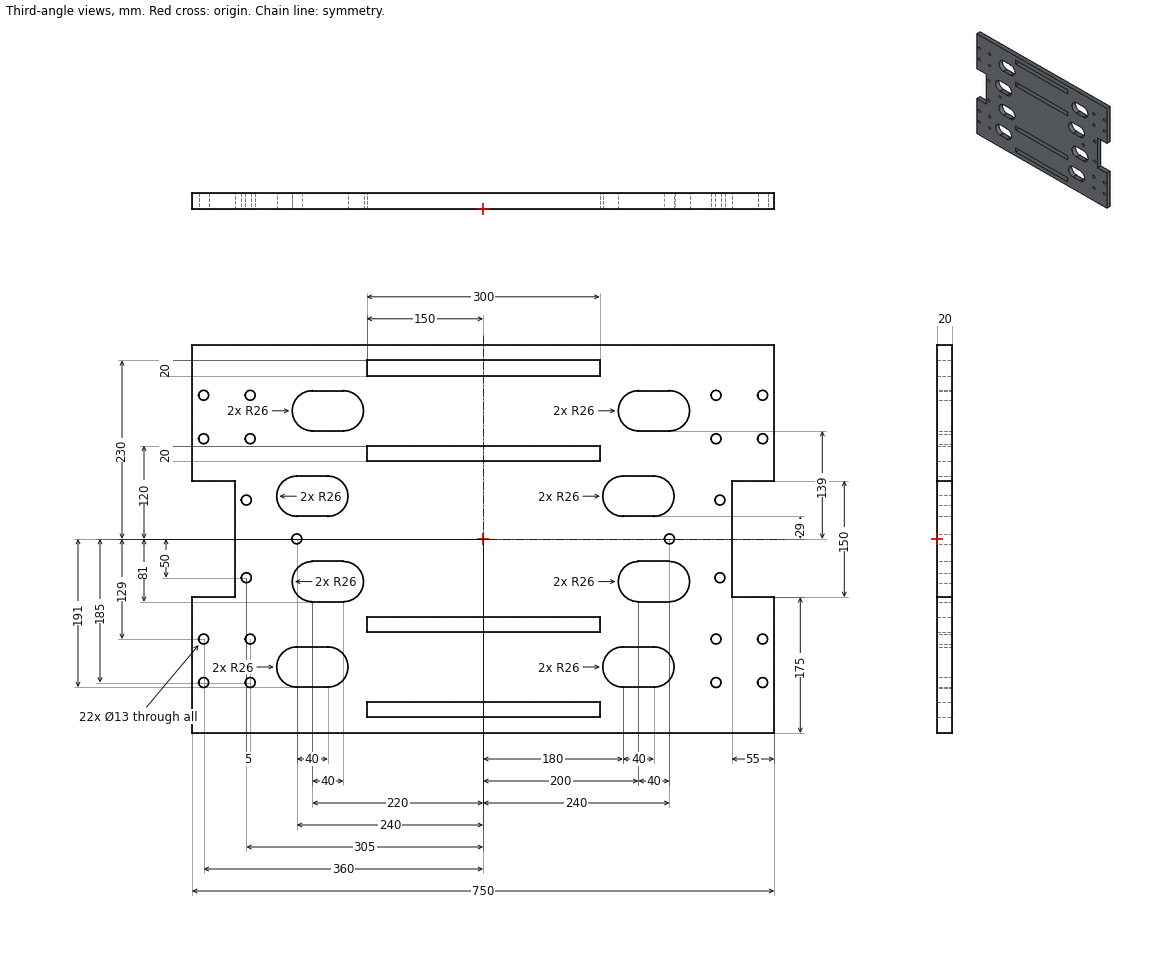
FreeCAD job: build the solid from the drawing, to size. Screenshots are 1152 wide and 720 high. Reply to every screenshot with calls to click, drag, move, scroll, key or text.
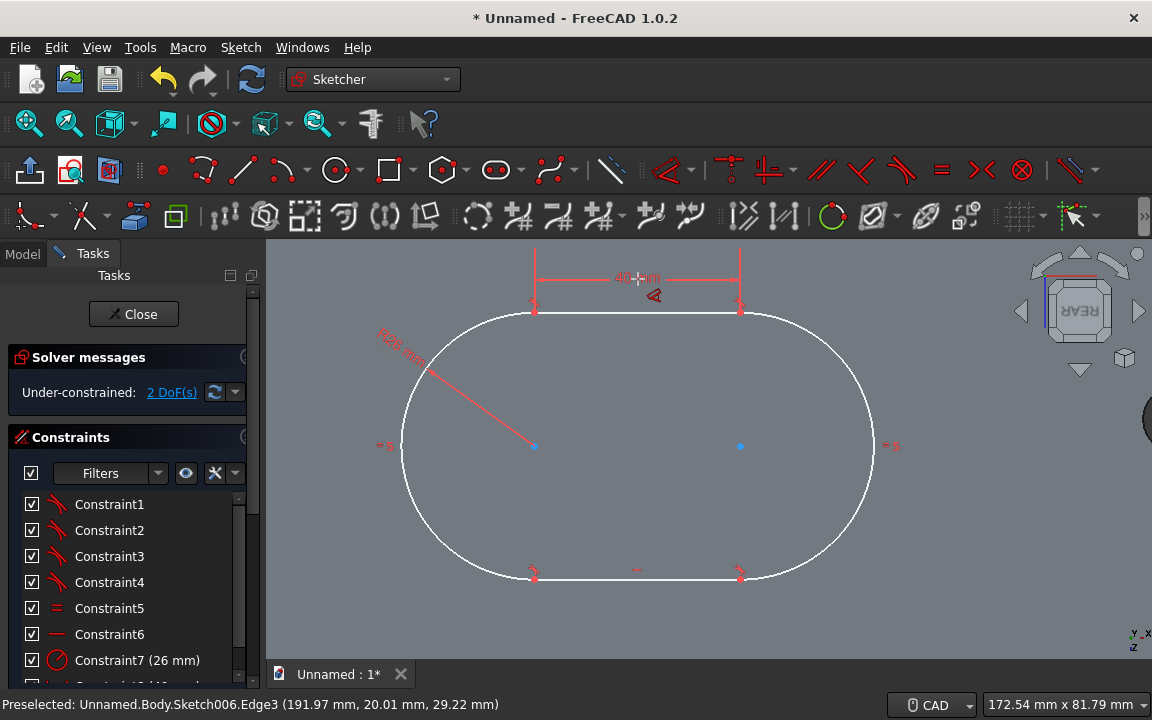
click(535, 313)
click(715, 290)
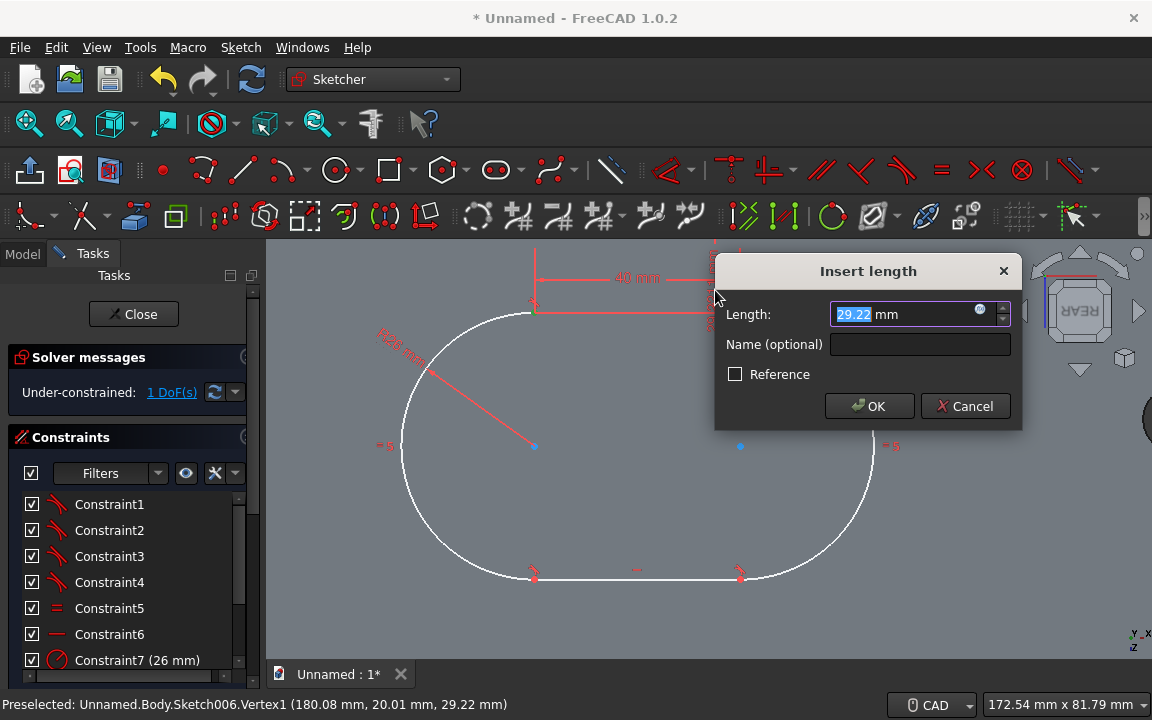
text(29)
key(Return)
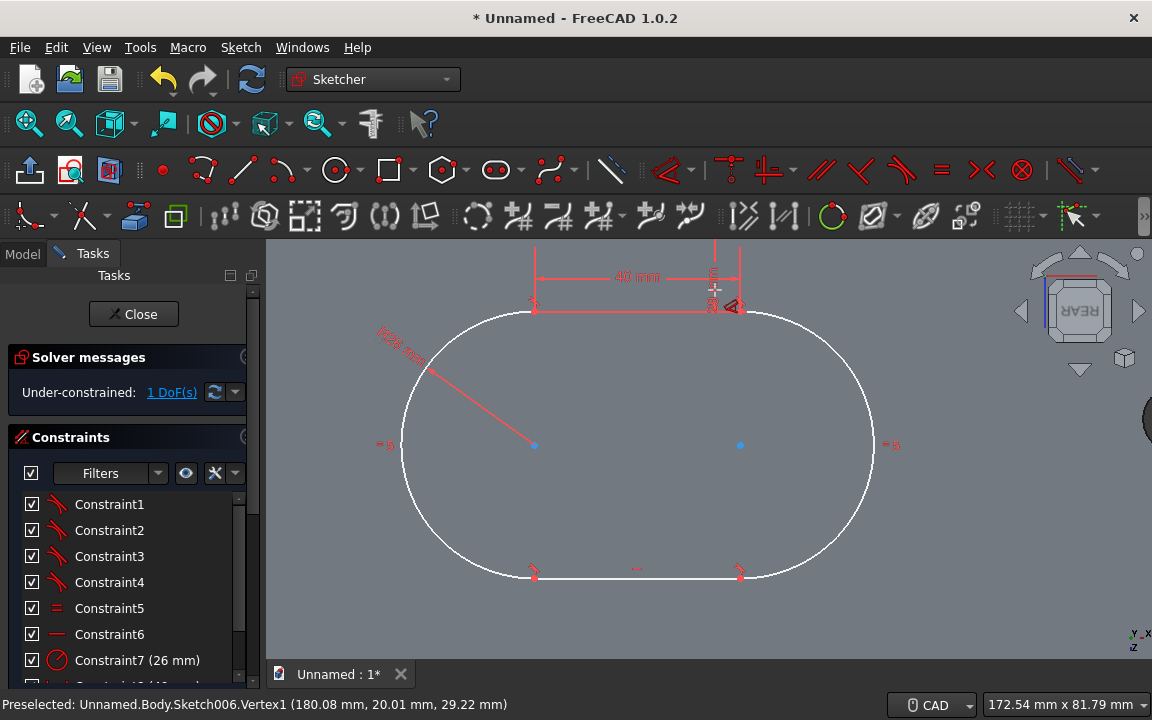
click(535, 312)
click(330, 346)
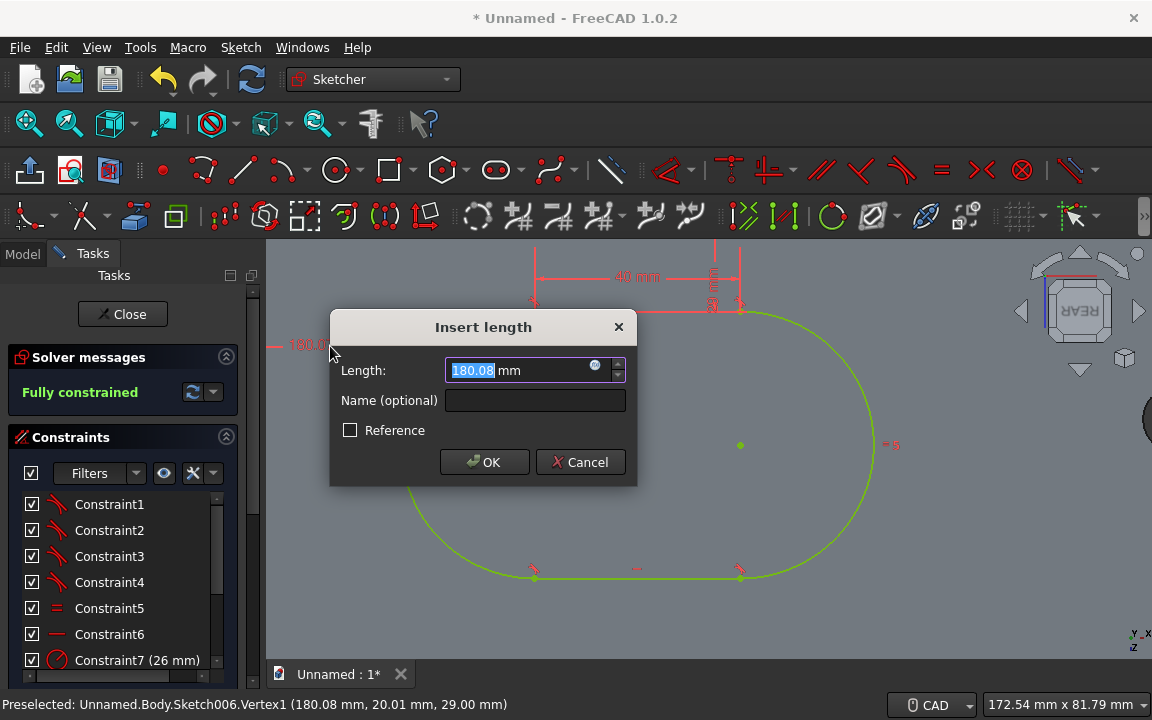
text(180)
key(Return)
key(Escape)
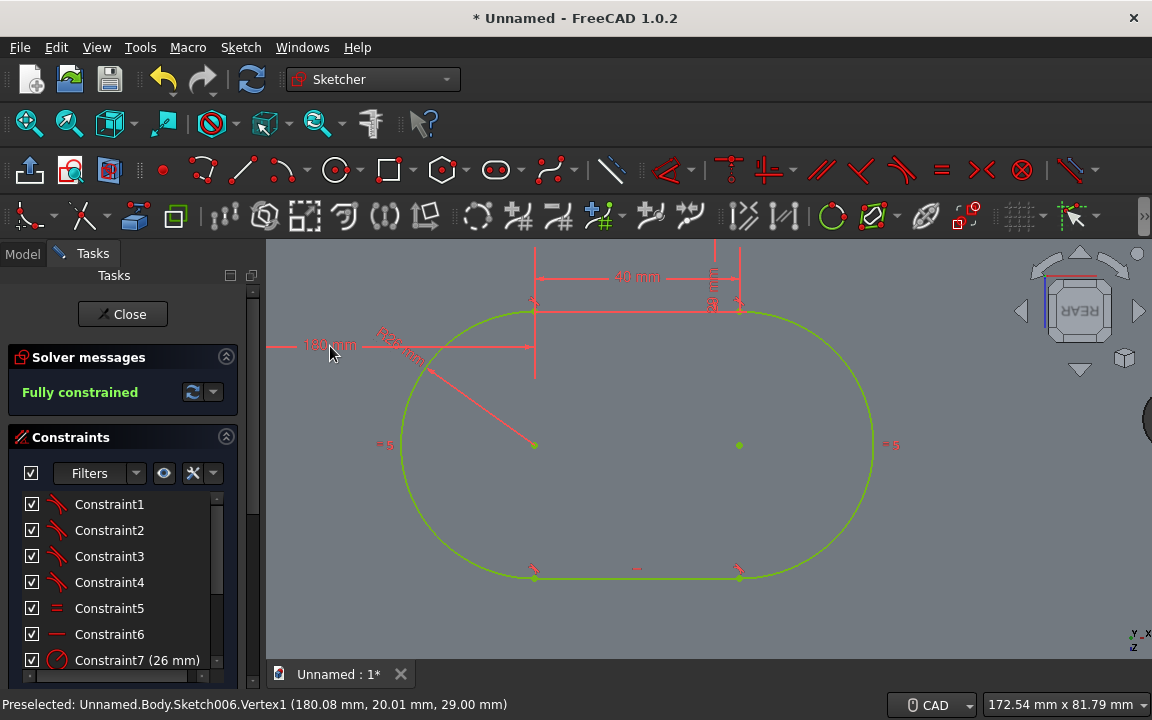
click(123, 314)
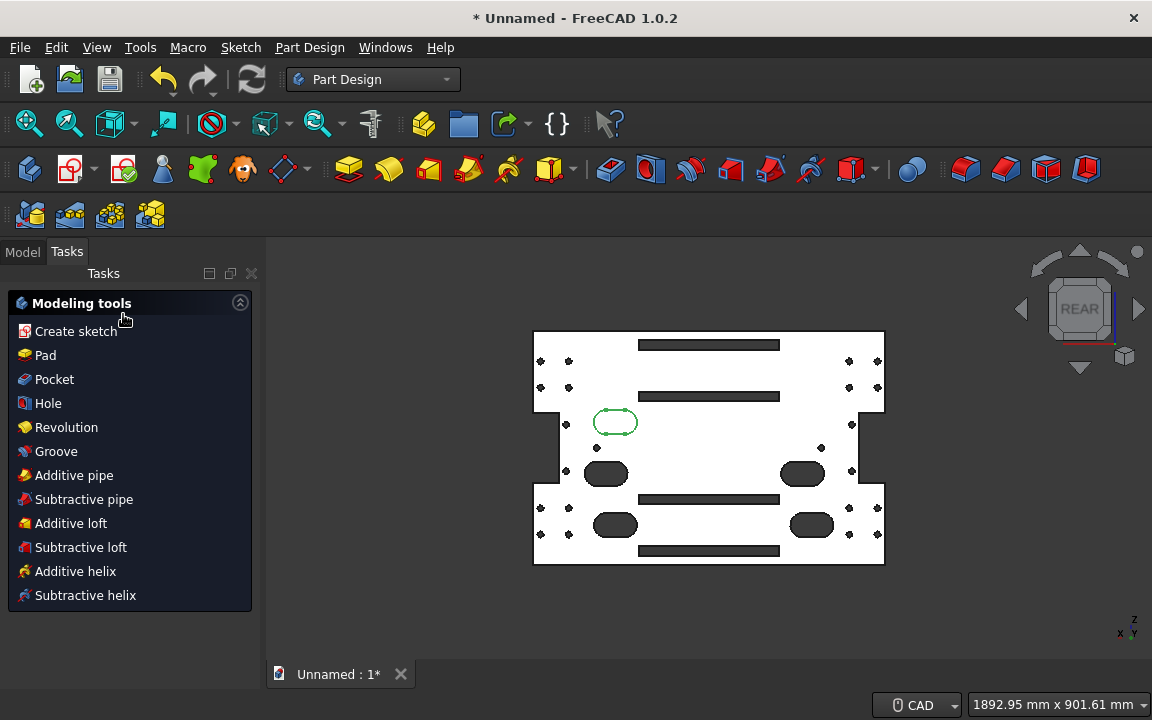
click(612, 170)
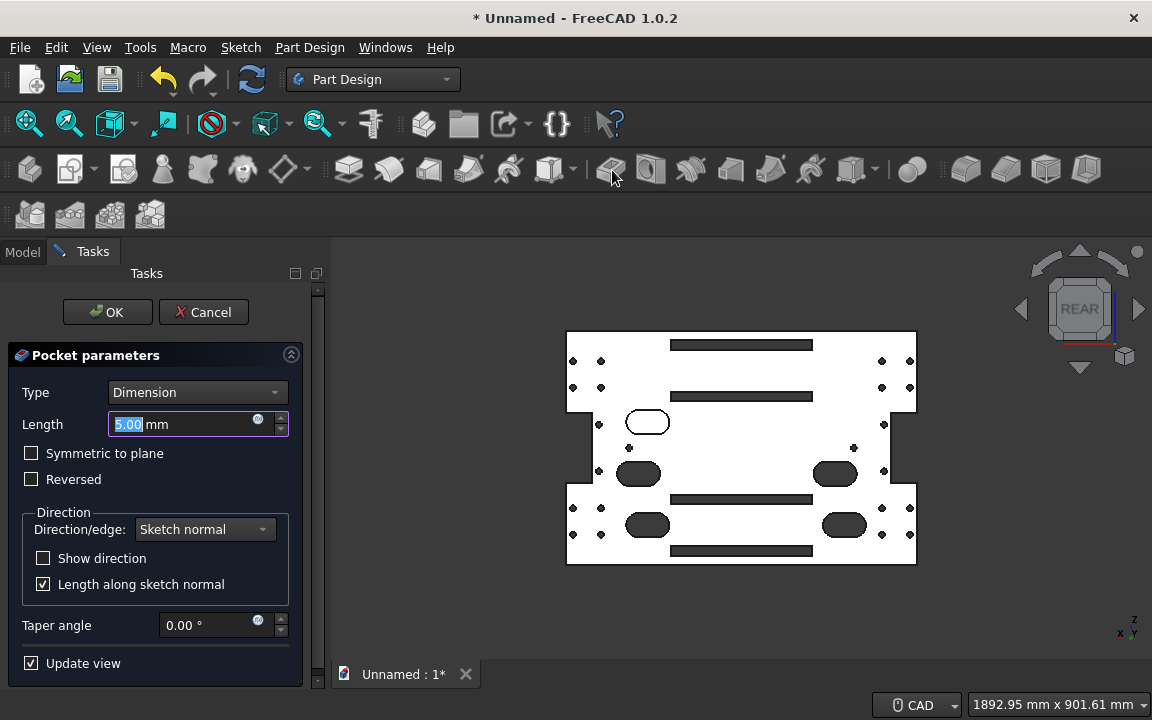
click(198, 392)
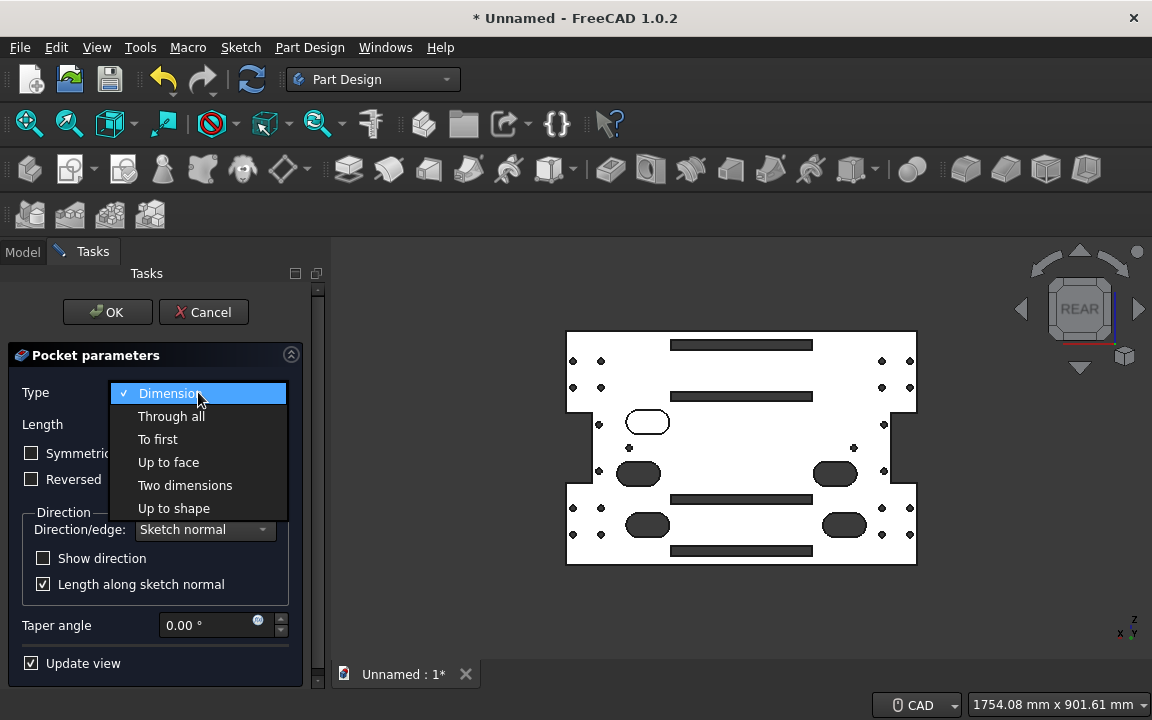
click(198, 440)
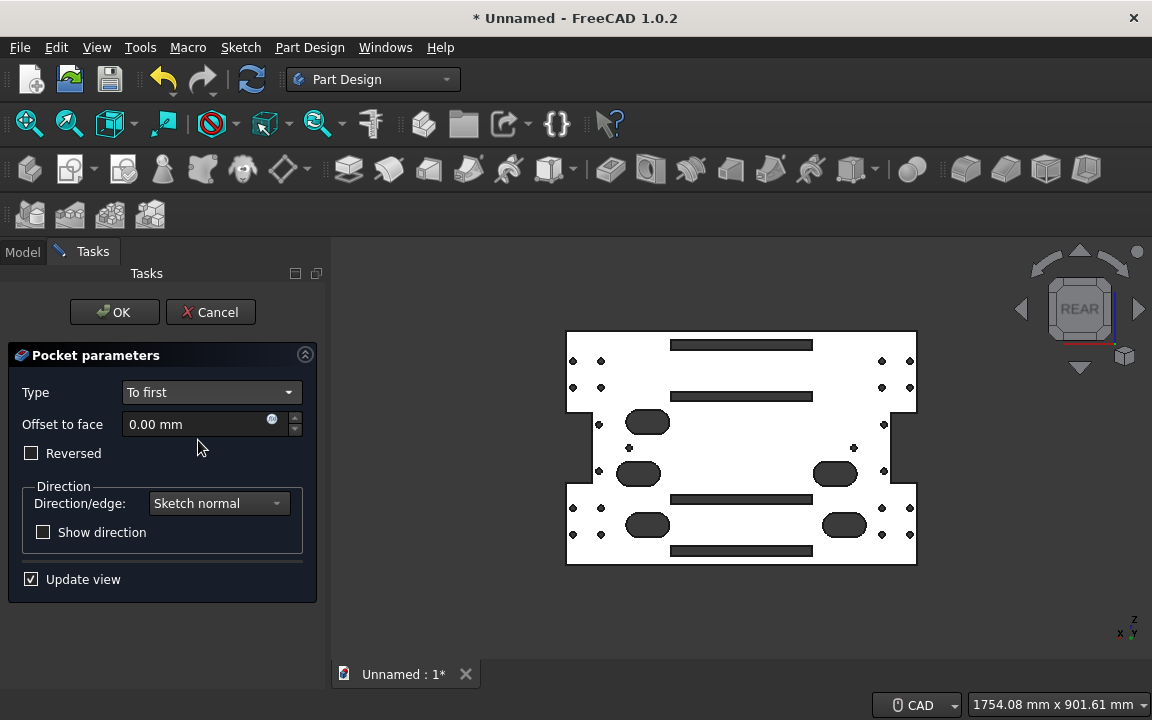
click(115, 312)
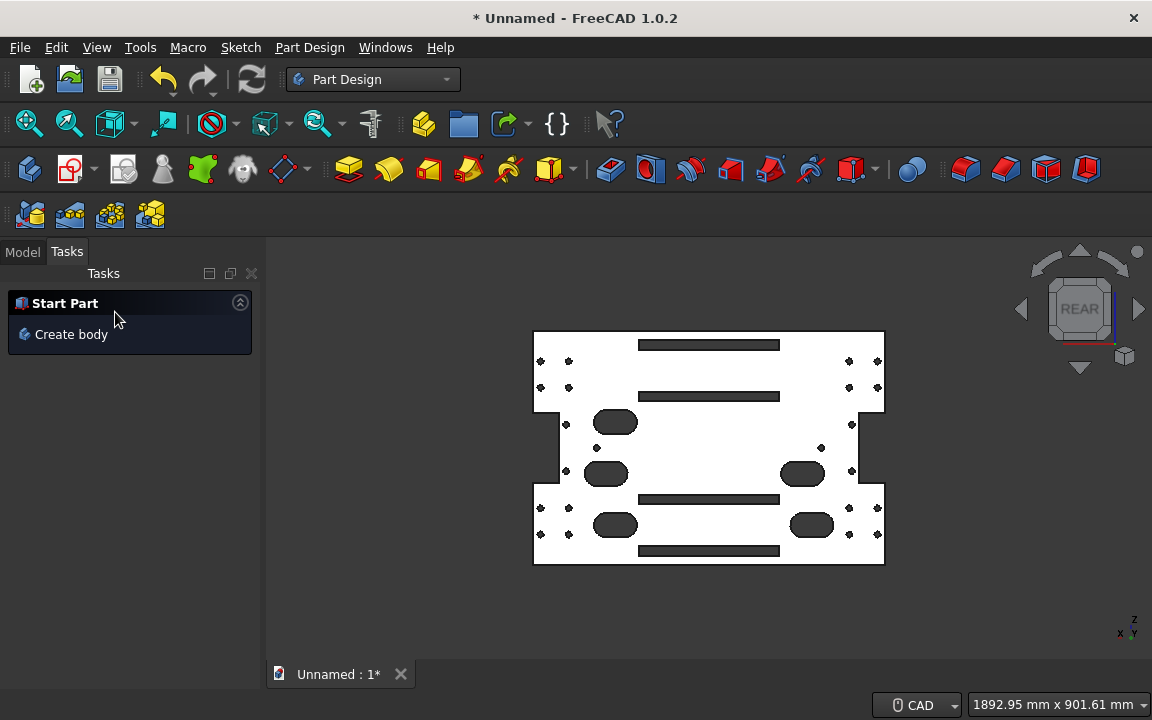
click(709, 447)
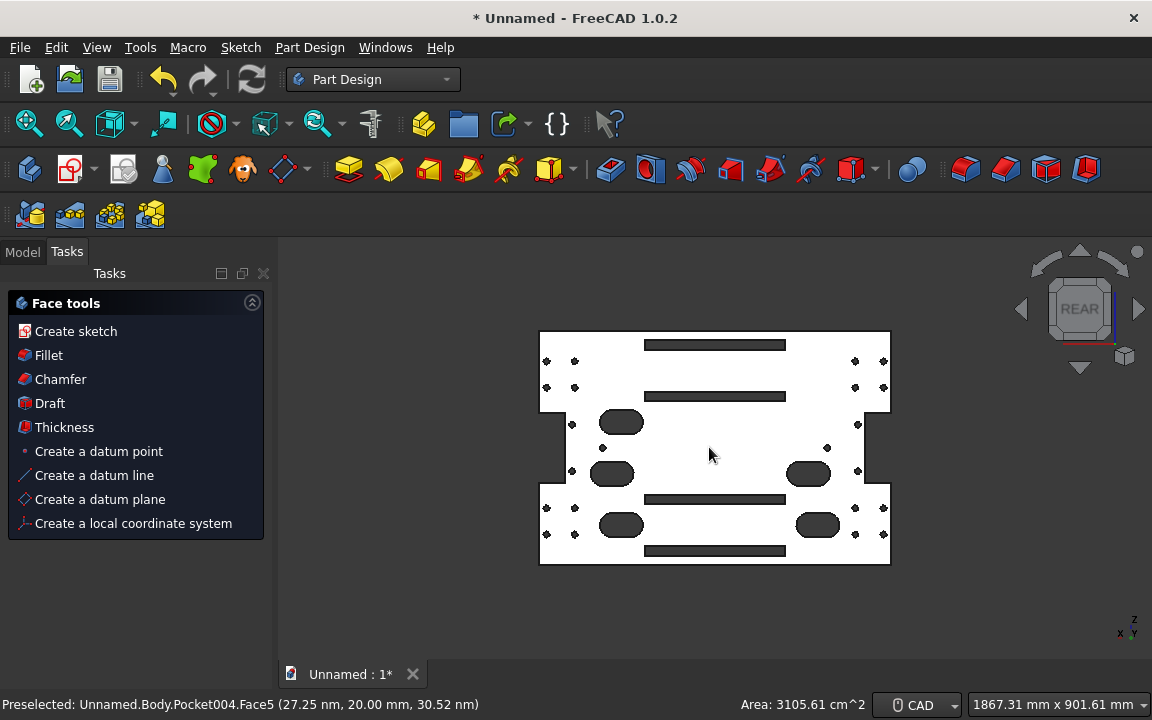
click(70, 170)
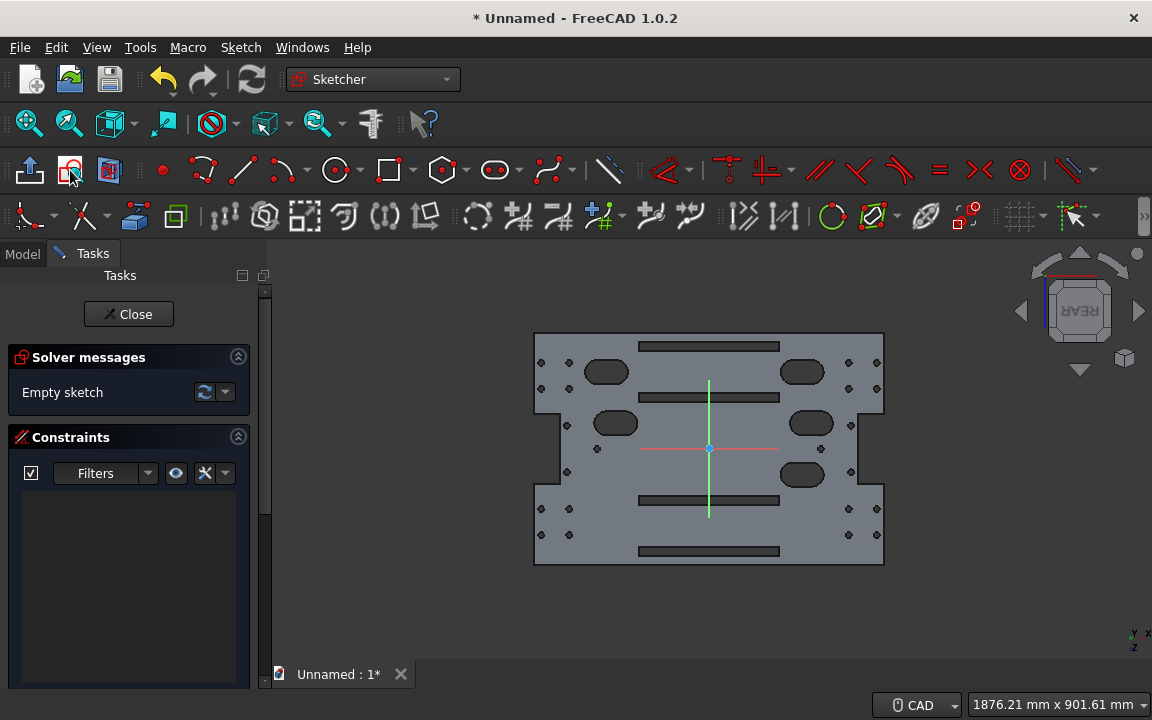
scroll(829, 534, up, 12)